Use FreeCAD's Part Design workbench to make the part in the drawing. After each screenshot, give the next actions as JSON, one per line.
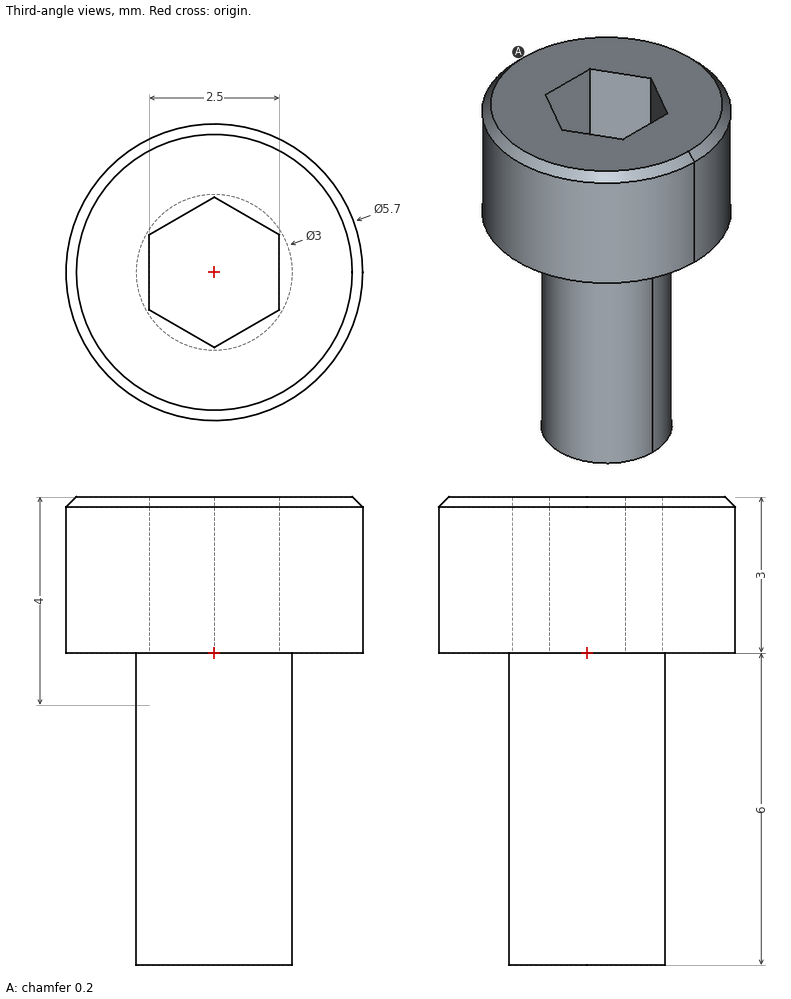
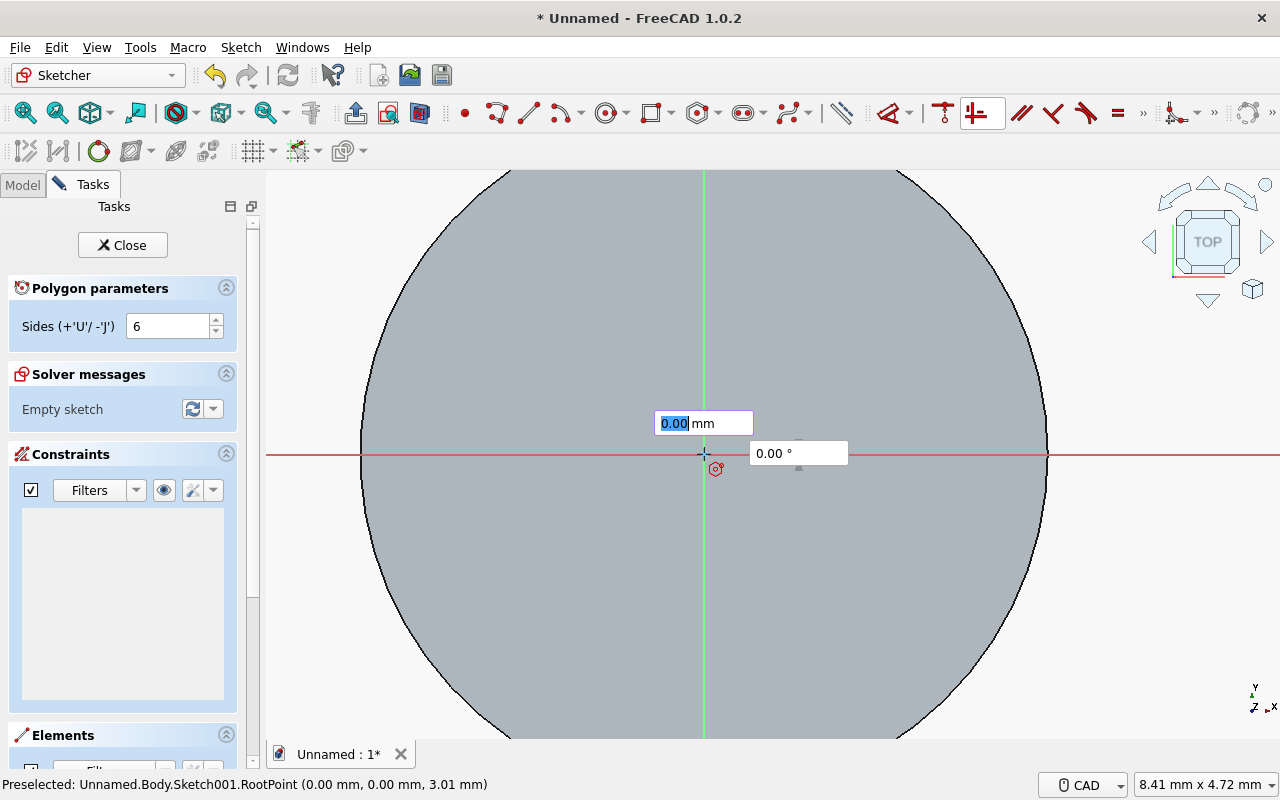
{"action": "left_click", "coordinate": [704, 280]}
{"action": "right_click", "coordinate": [704, 280]}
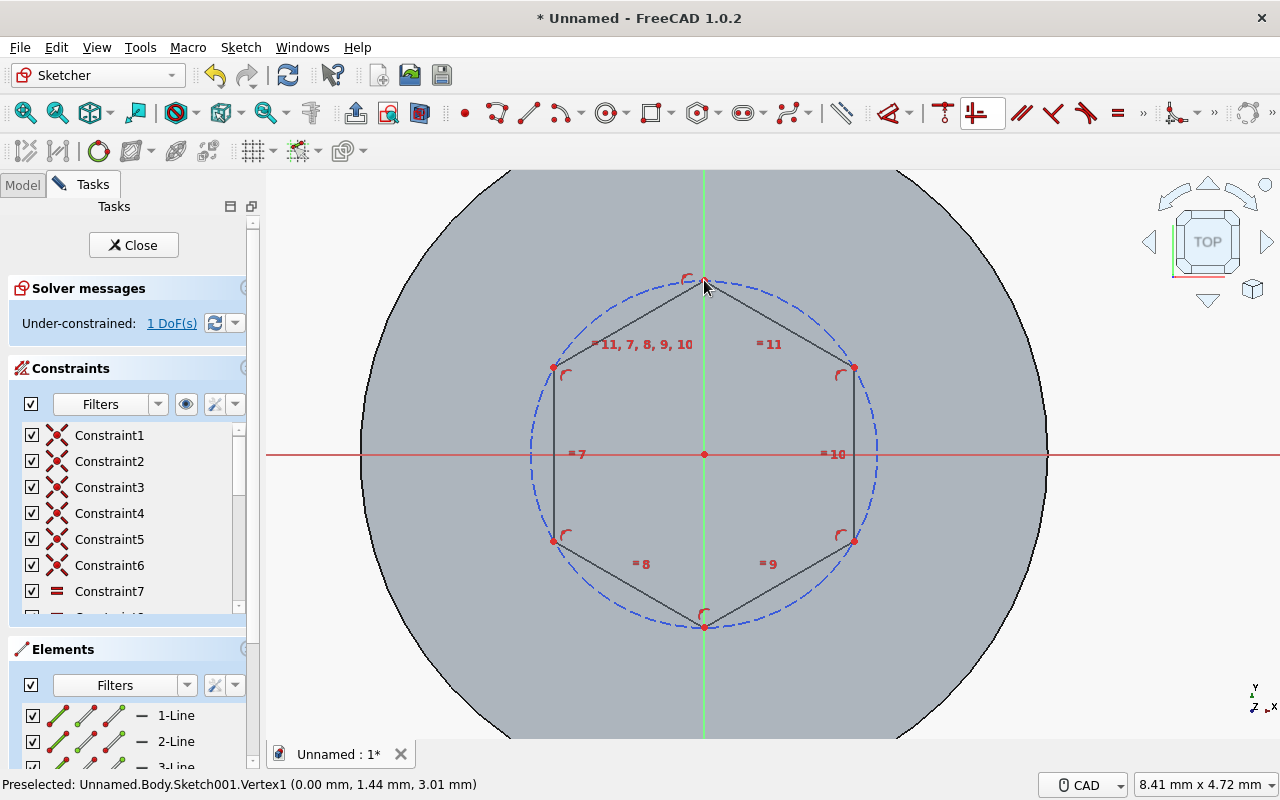
{"action": "left_click", "coordinate": [888, 114]}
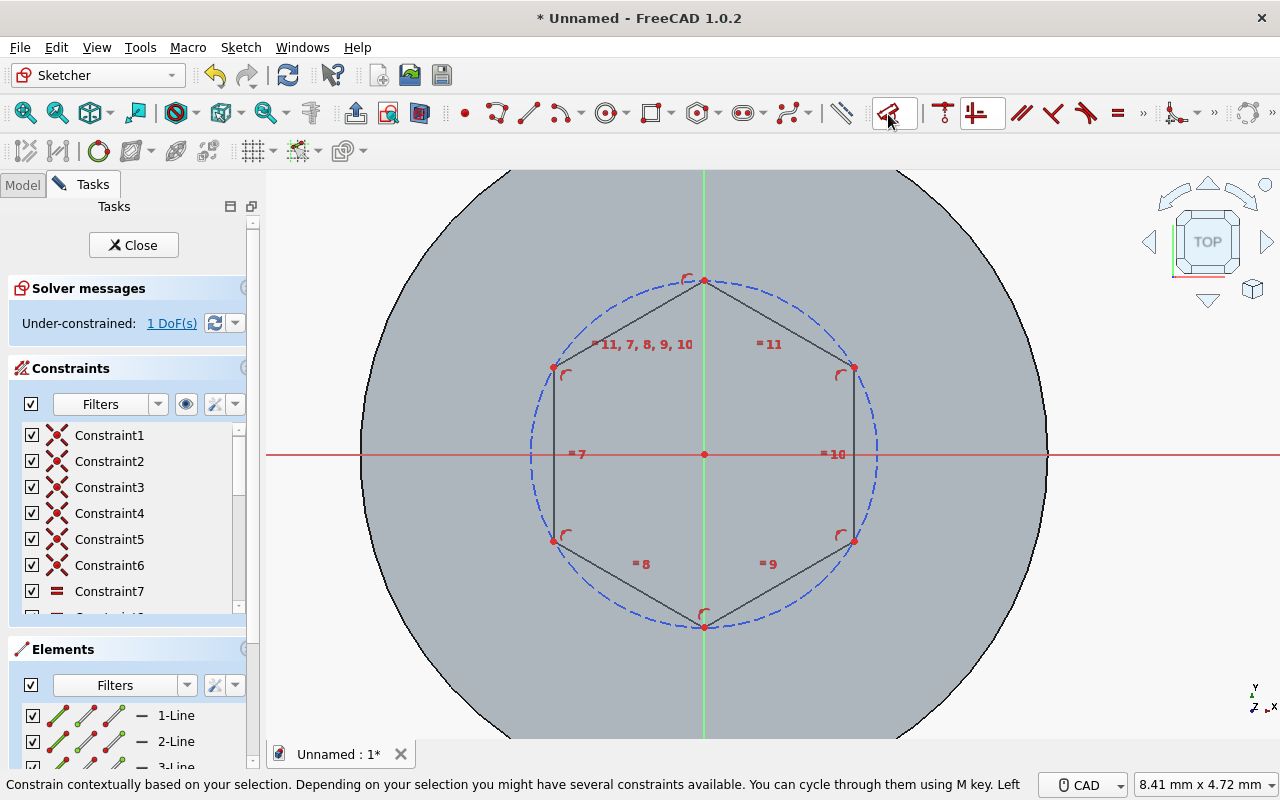
{"action": "left_click", "coordinate": [554, 368]}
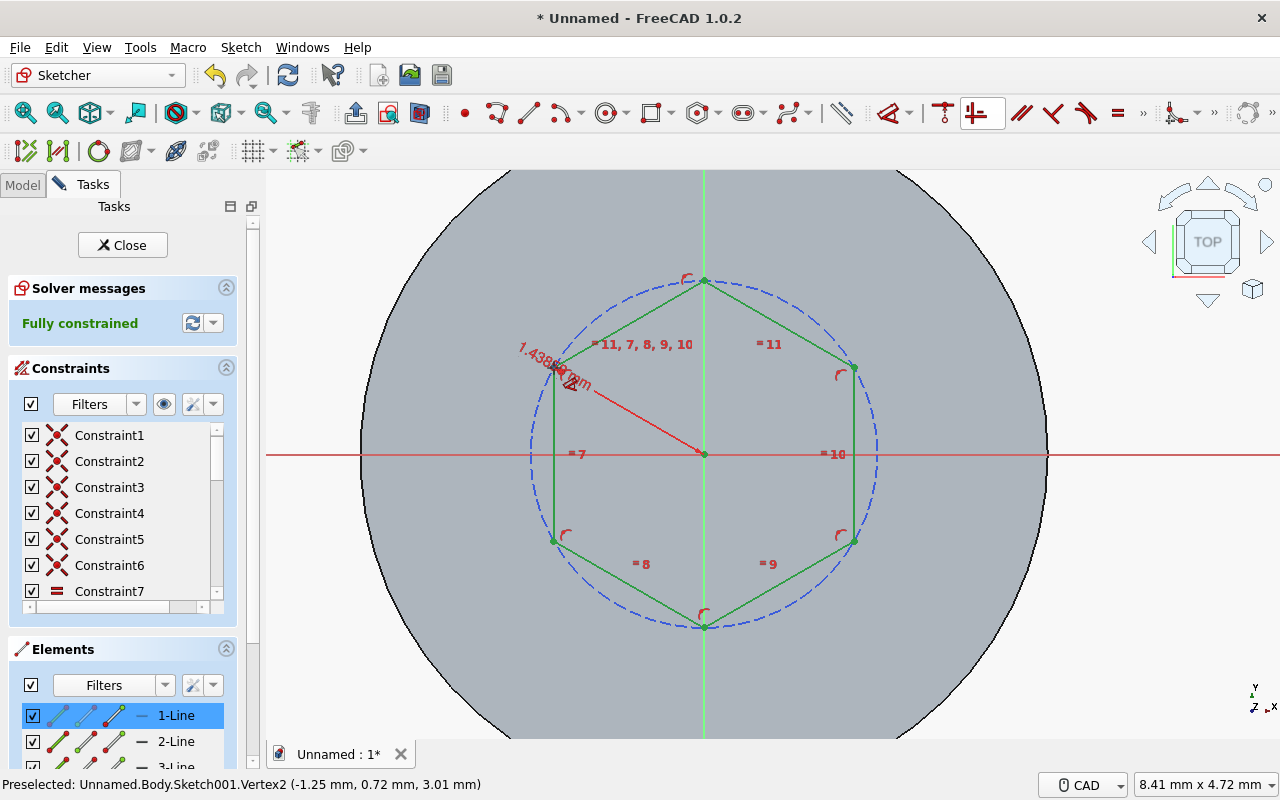
{"action": "left_click", "coordinate": [854, 541]}
{"action": "left_click", "coordinate": [599, 623]}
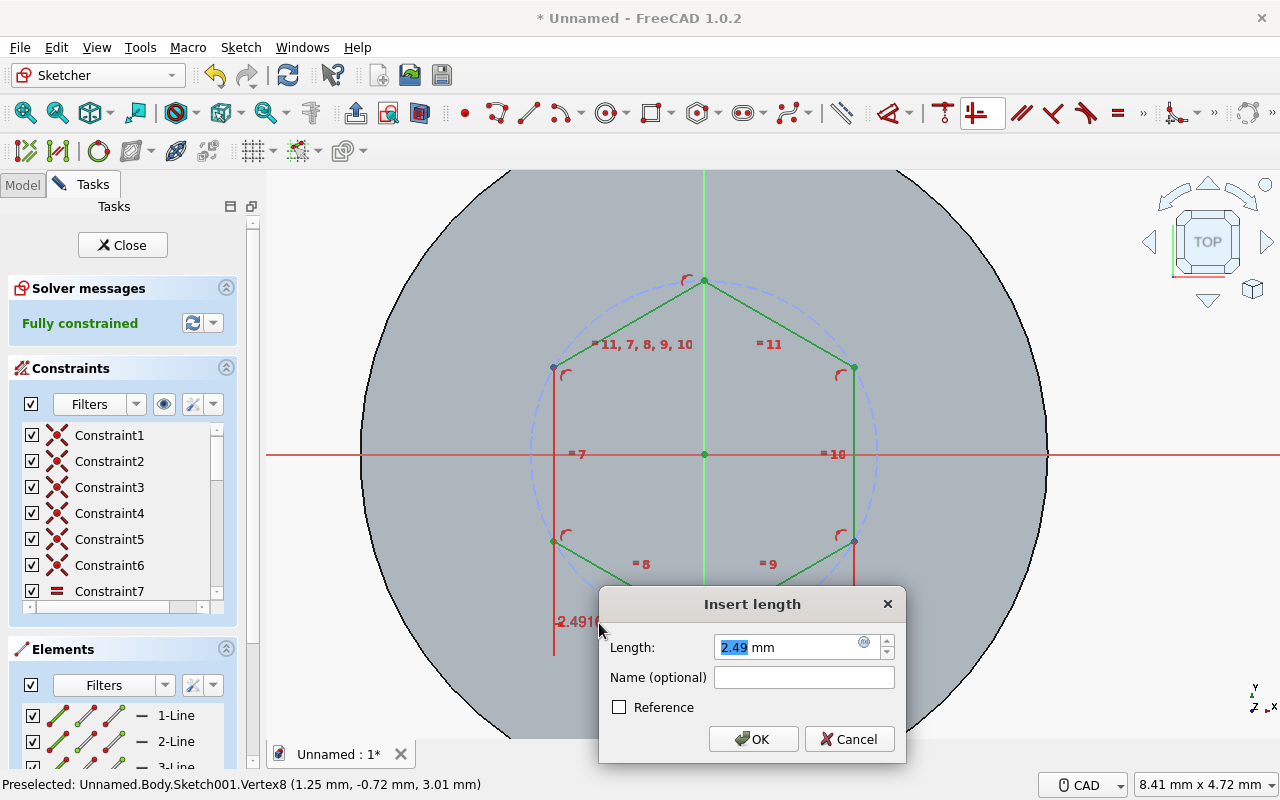
{"action": "type", "text": "2.5"}
{"action": "key", "text": "Return"}
{"action": "key", "text": "Escape"}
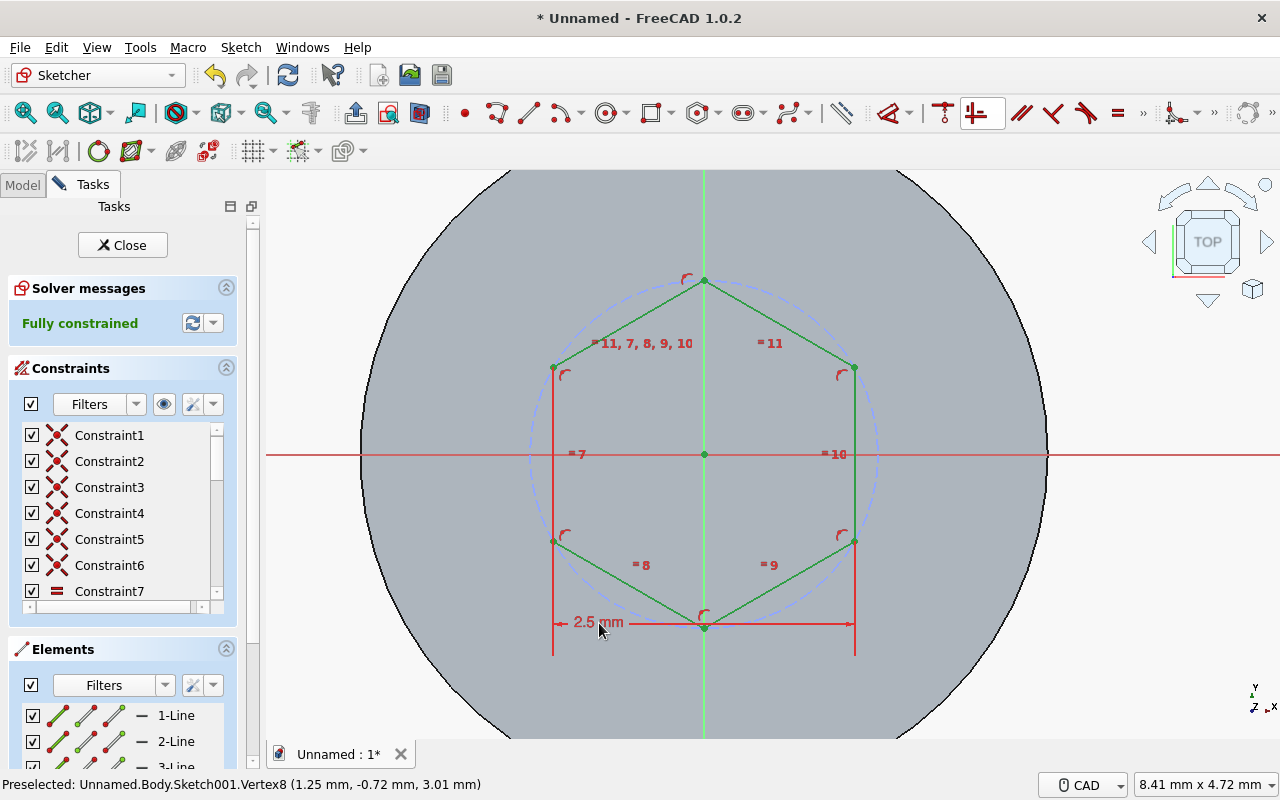
{"action": "left_click", "coordinate": [123, 245]}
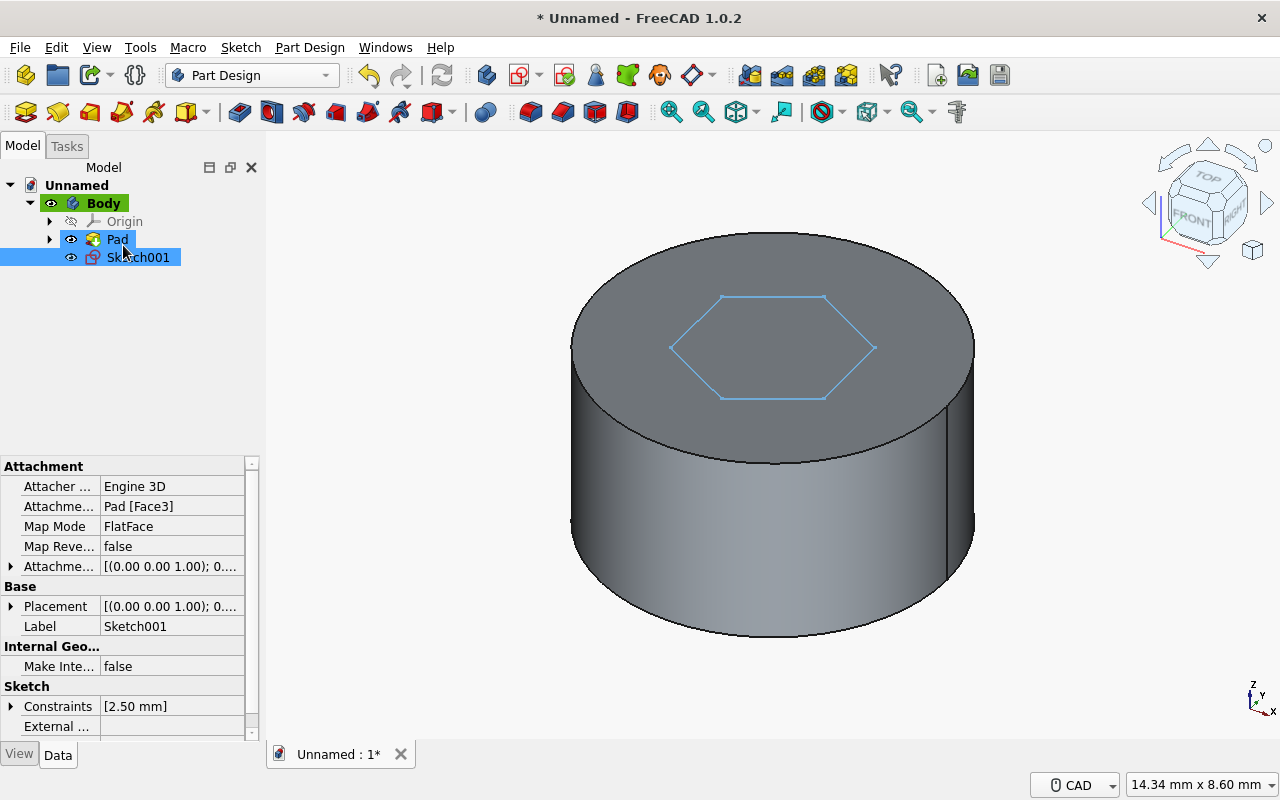
{"action": "left_click", "coordinate": [240, 112]}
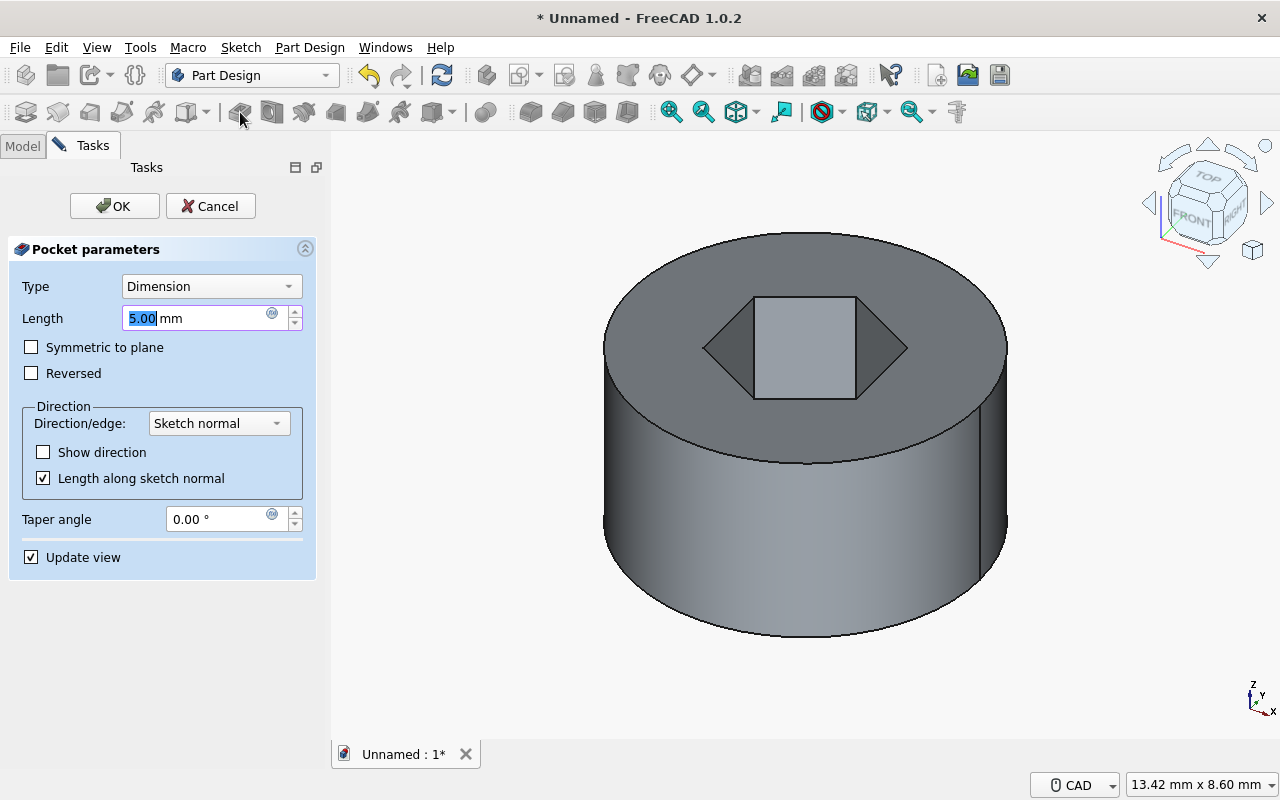
{"action": "type", "text": "4"}
{"action": "key", "text": "Tab"}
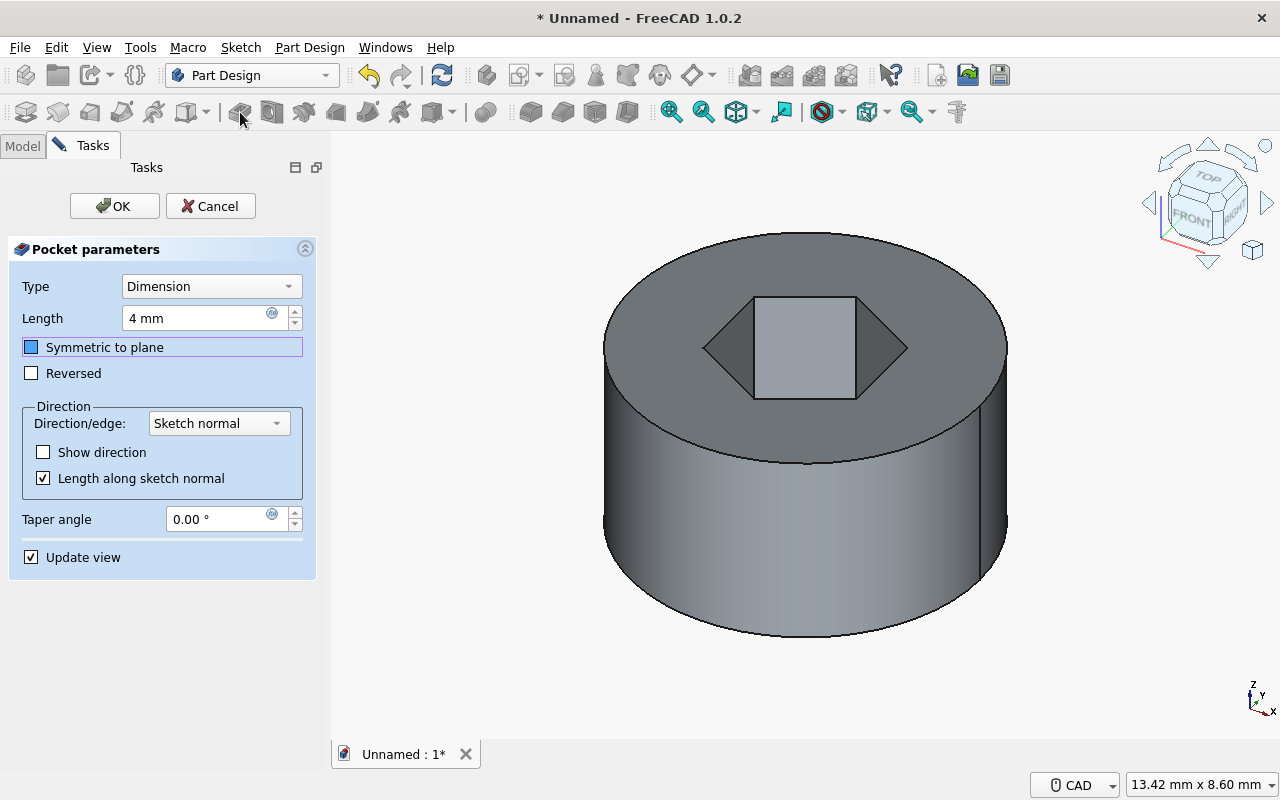
{"action": "left_click", "coordinate": [115, 206]}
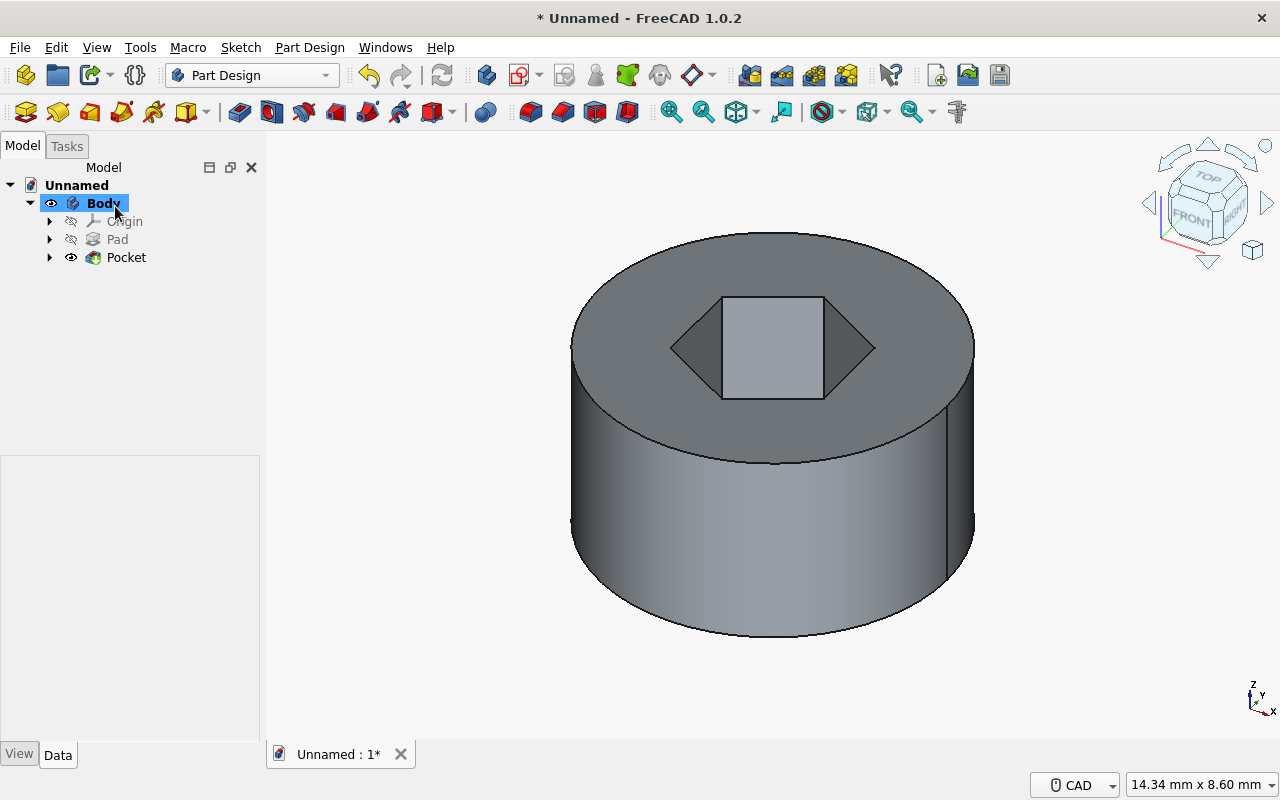
{"action": "left_click", "coordinate": [572, 359]}